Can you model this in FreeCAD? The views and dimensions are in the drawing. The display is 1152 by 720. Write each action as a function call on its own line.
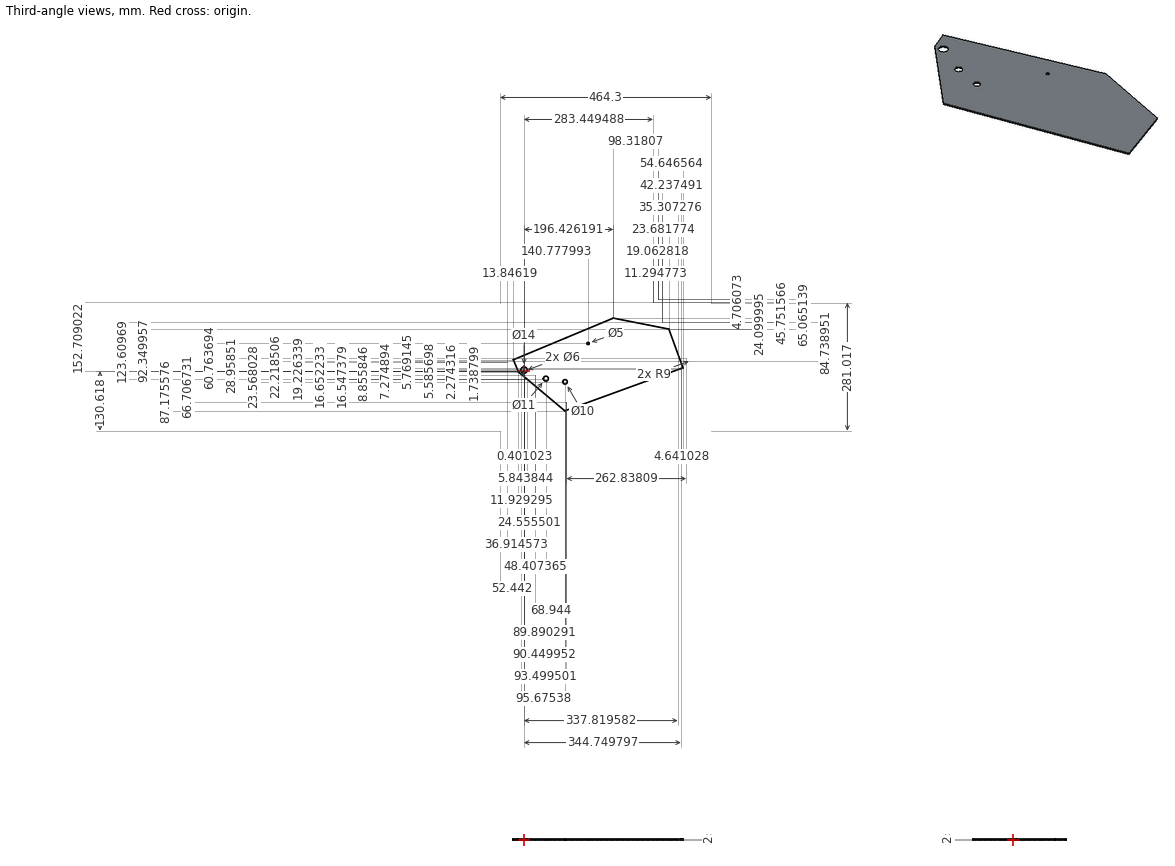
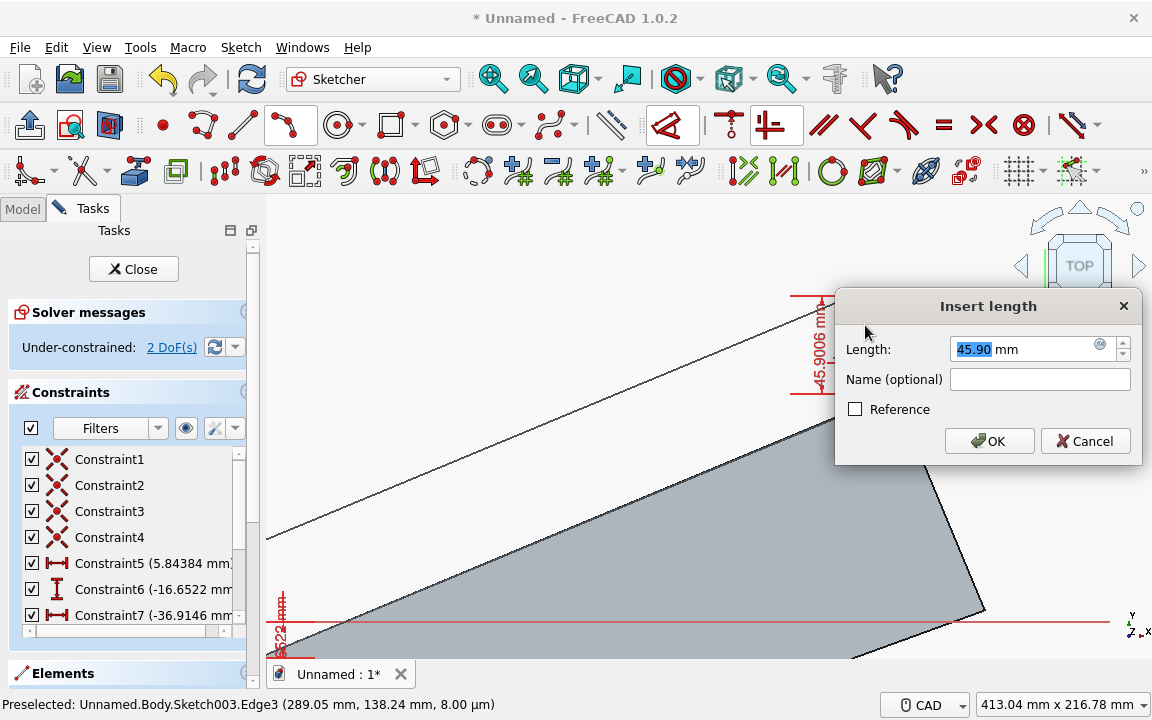
text(45.751566)
key(Return)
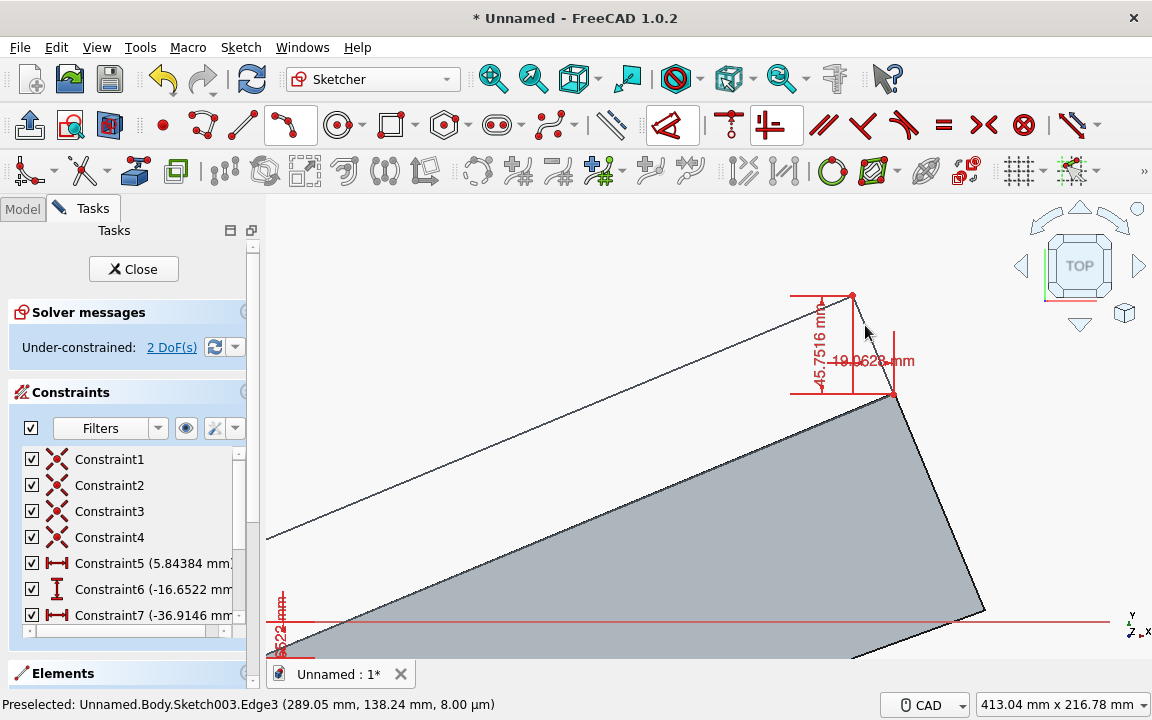
click(703, 473)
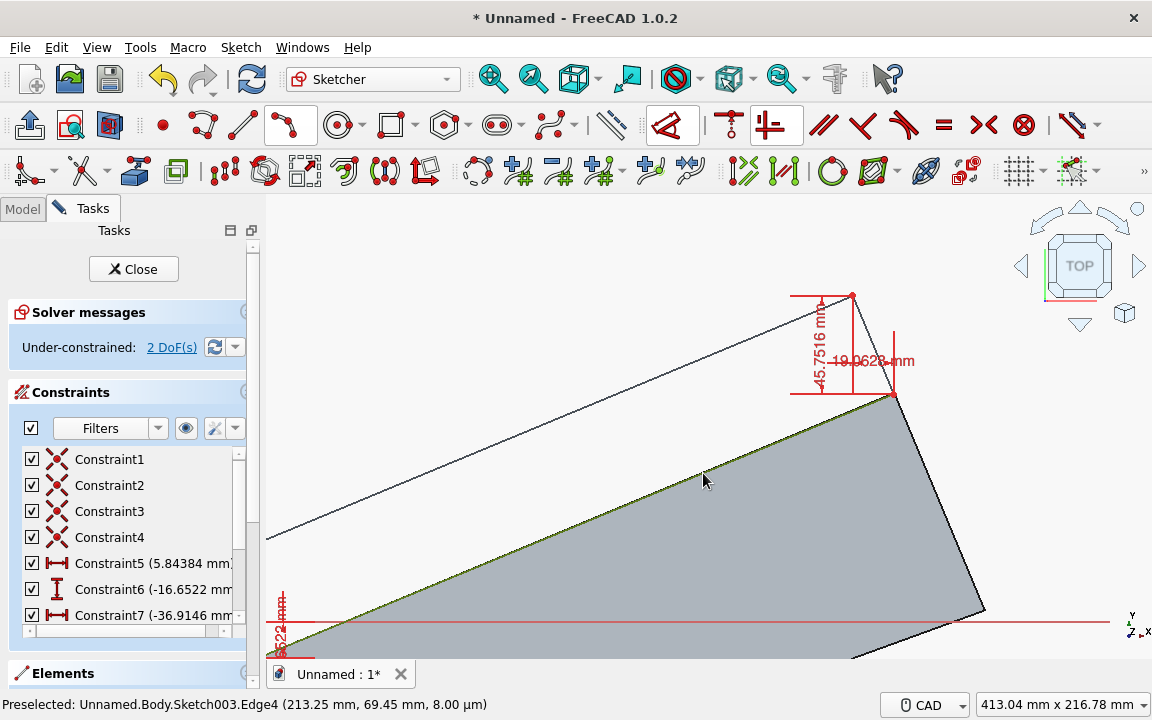
click(694, 126)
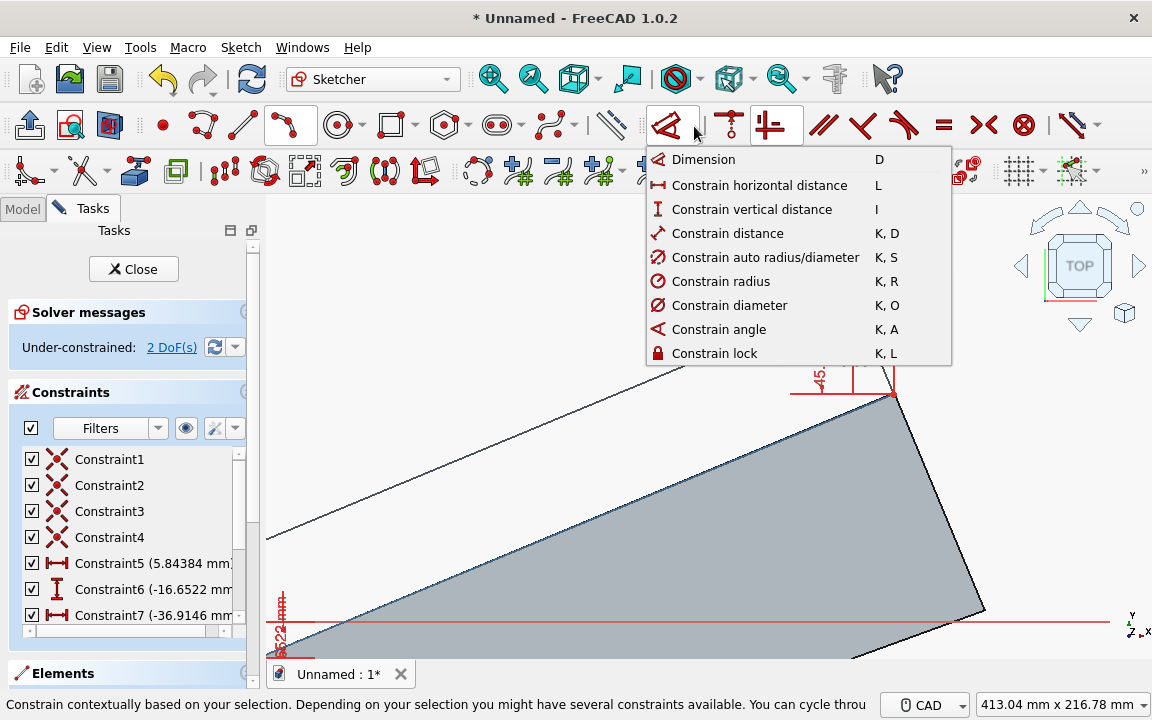
click(799, 209)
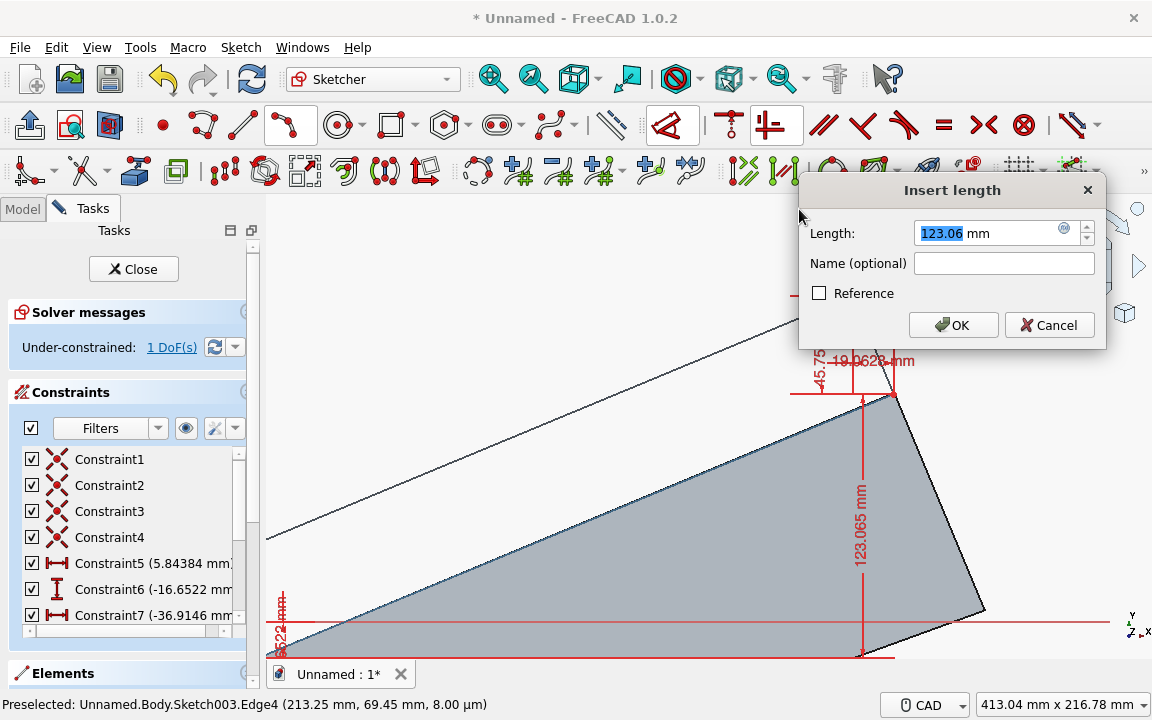
text(123.60969)
key(Return)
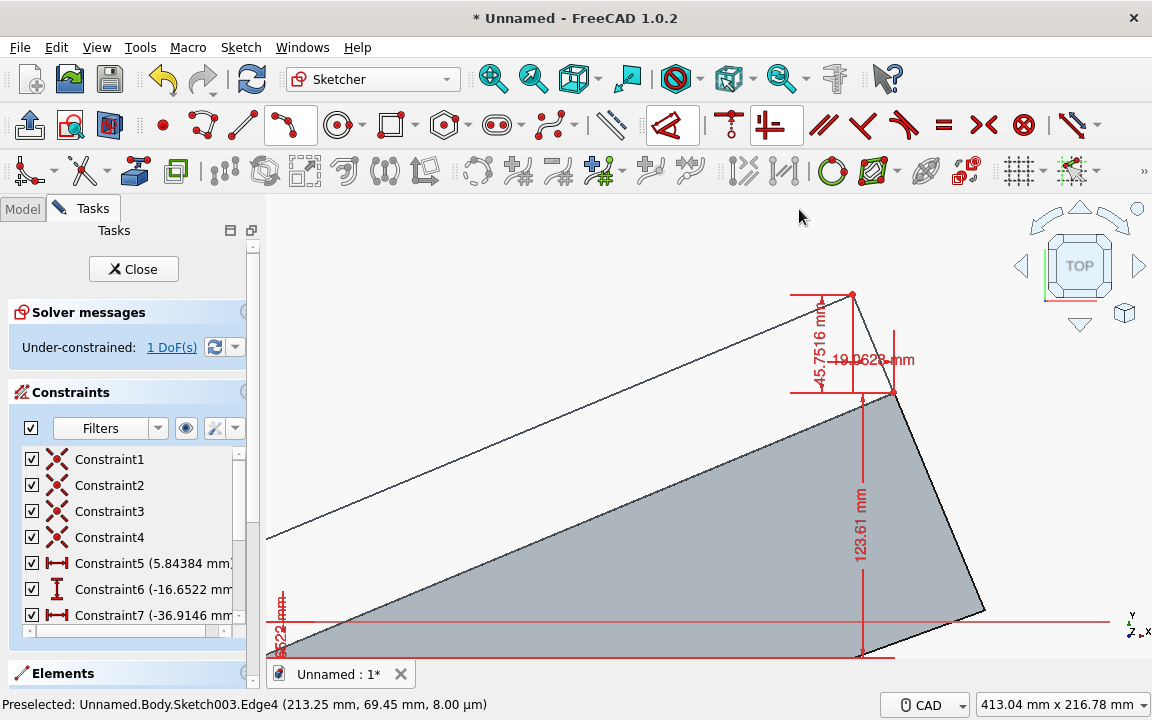
click(853, 295)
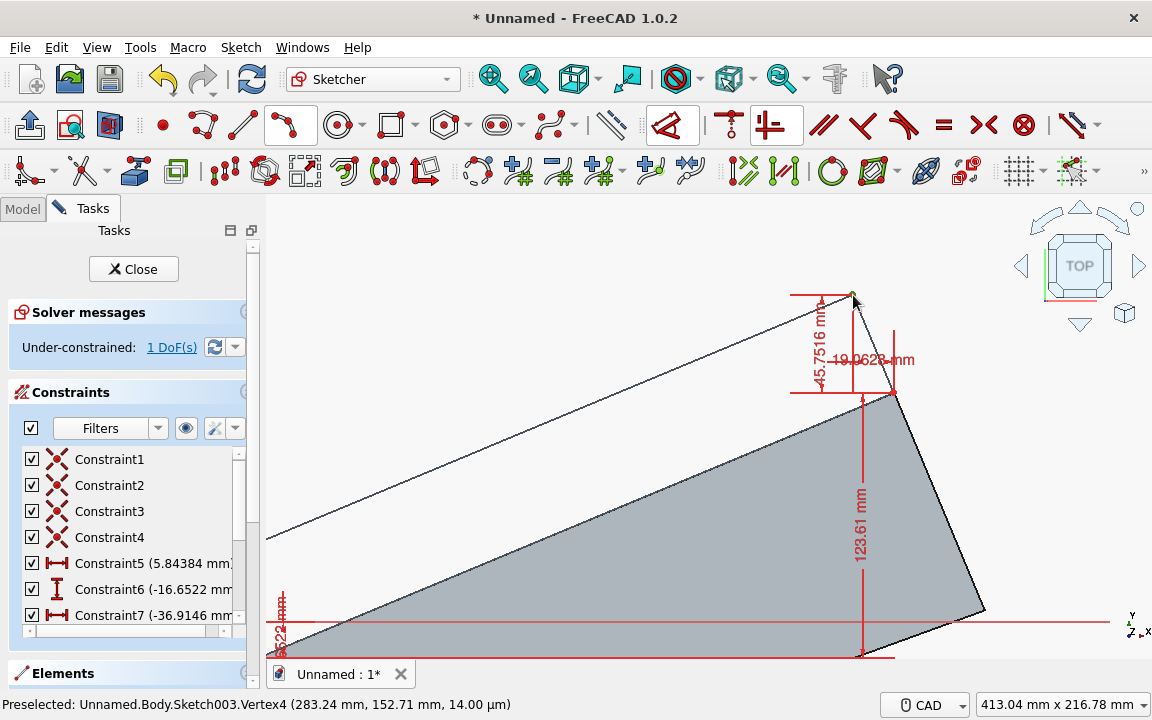
key(l)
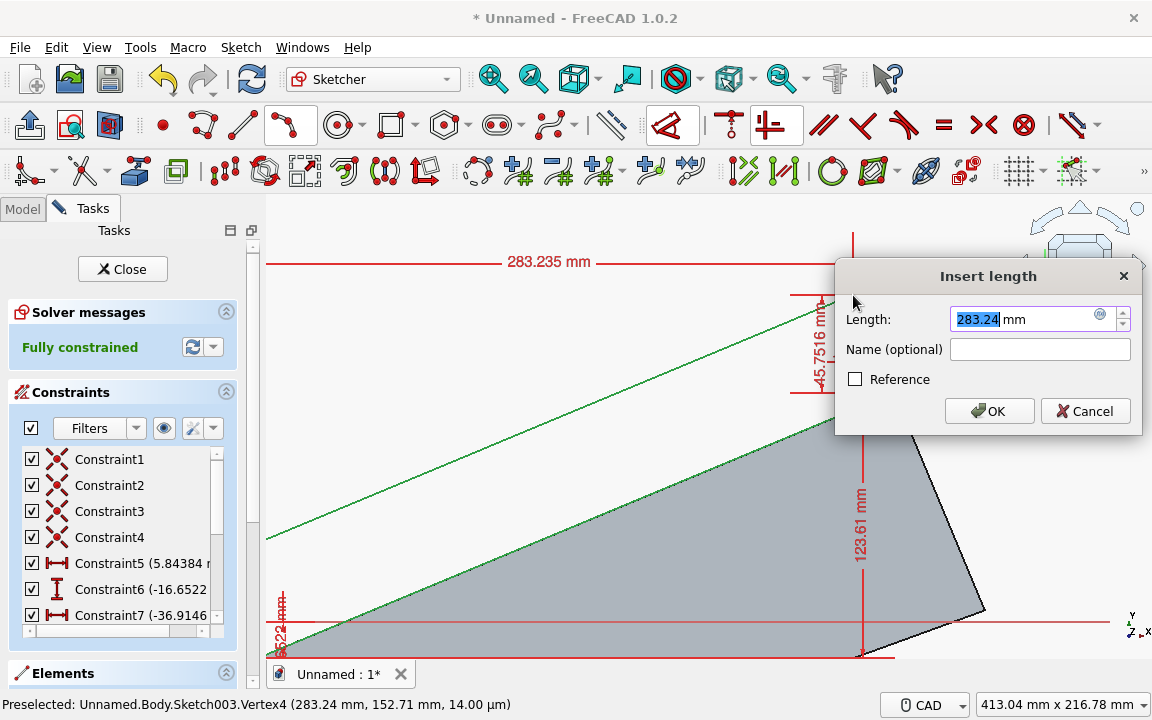
text(283.449488)
key(Return)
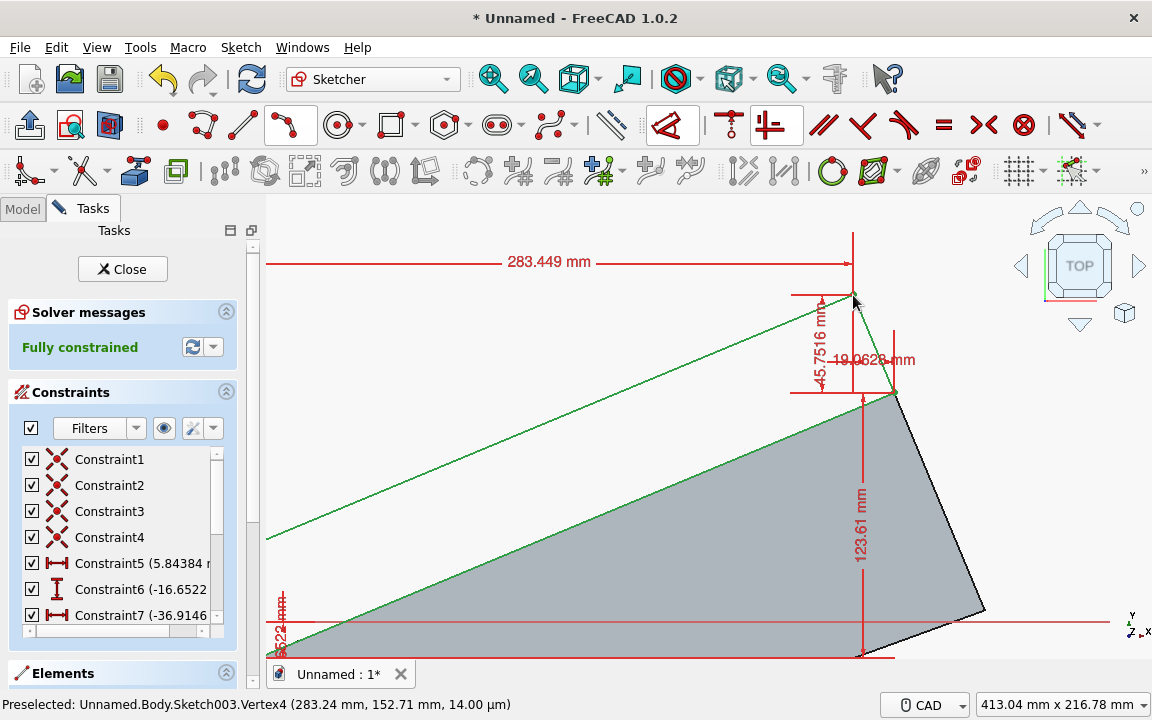
click(123, 269)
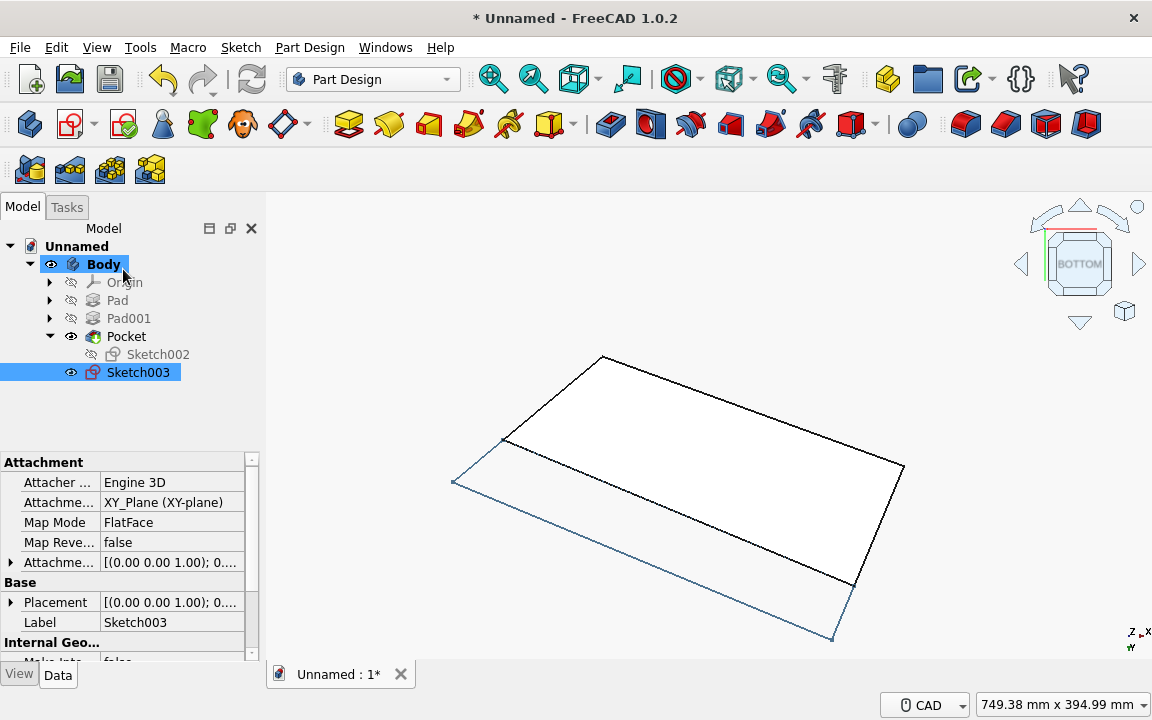
click(350, 124)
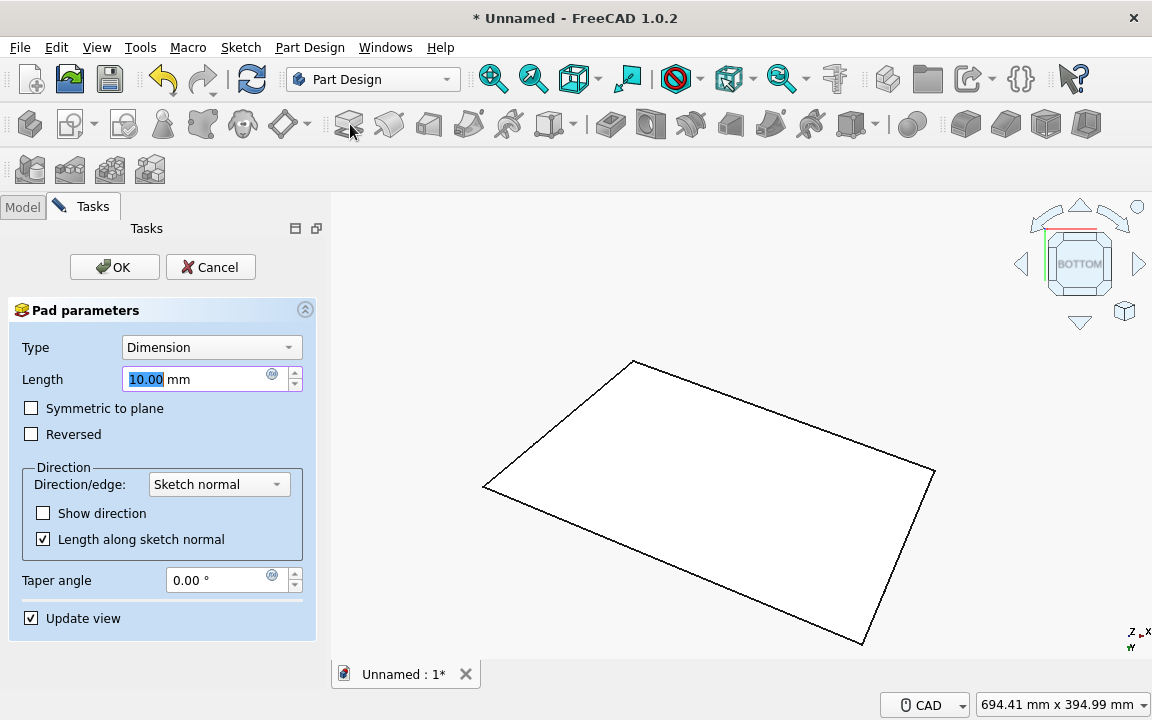
text(2)
key(Tab)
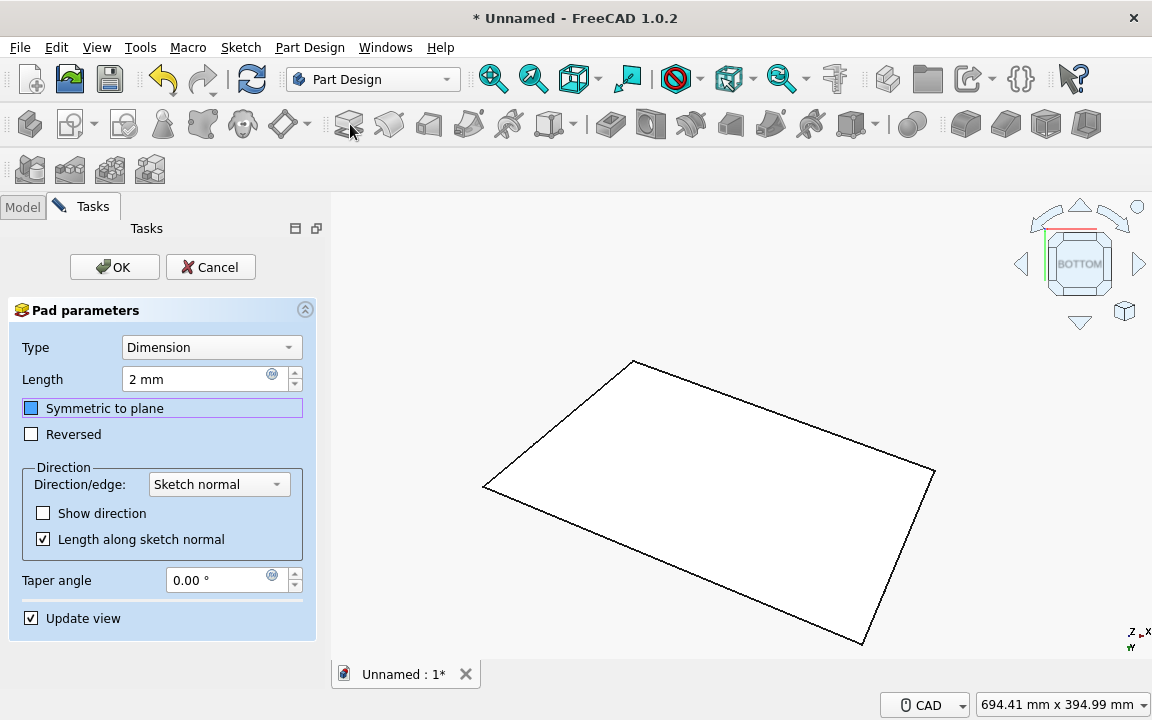
click(115, 267)